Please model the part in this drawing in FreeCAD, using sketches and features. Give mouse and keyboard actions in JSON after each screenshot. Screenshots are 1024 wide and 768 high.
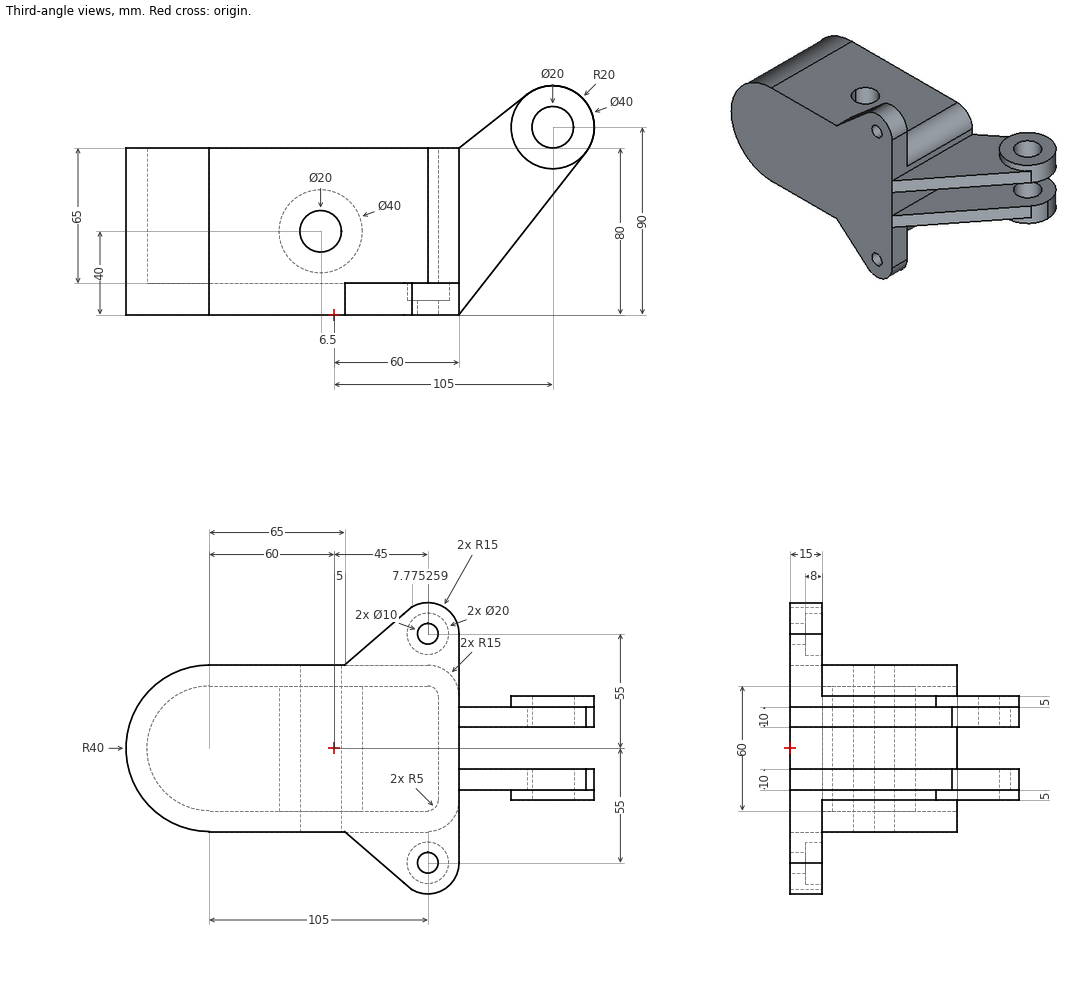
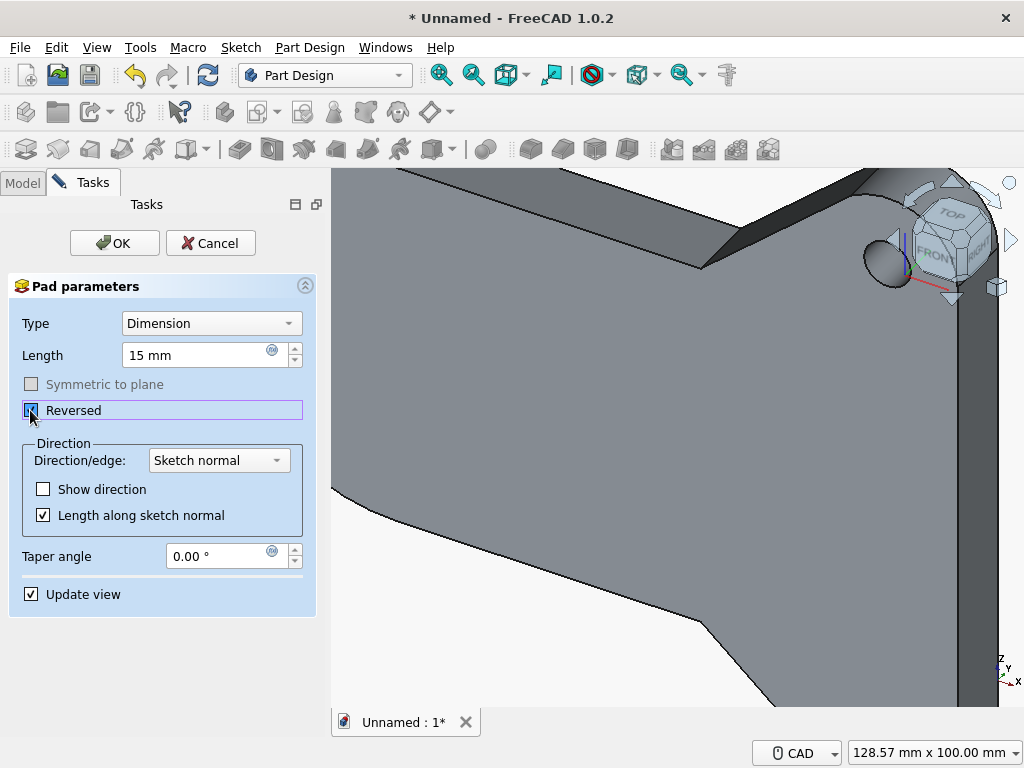
{"action": "left_click", "coordinate": [115, 243]}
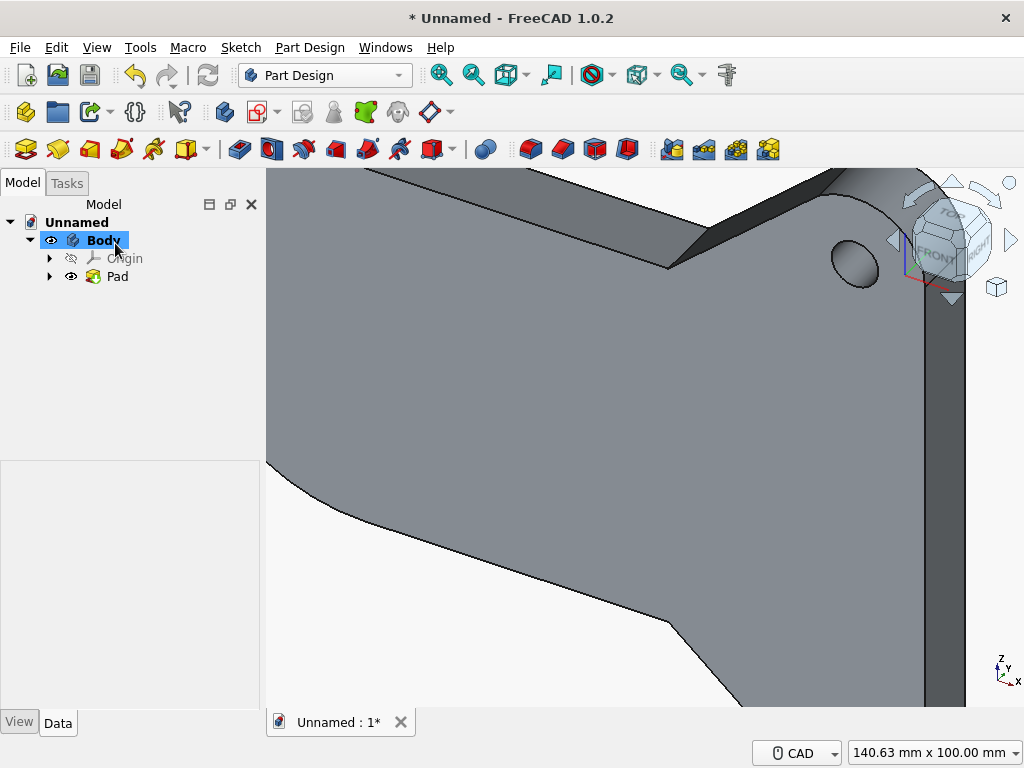
{"action": "left_click", "coordinate": [442, 76]}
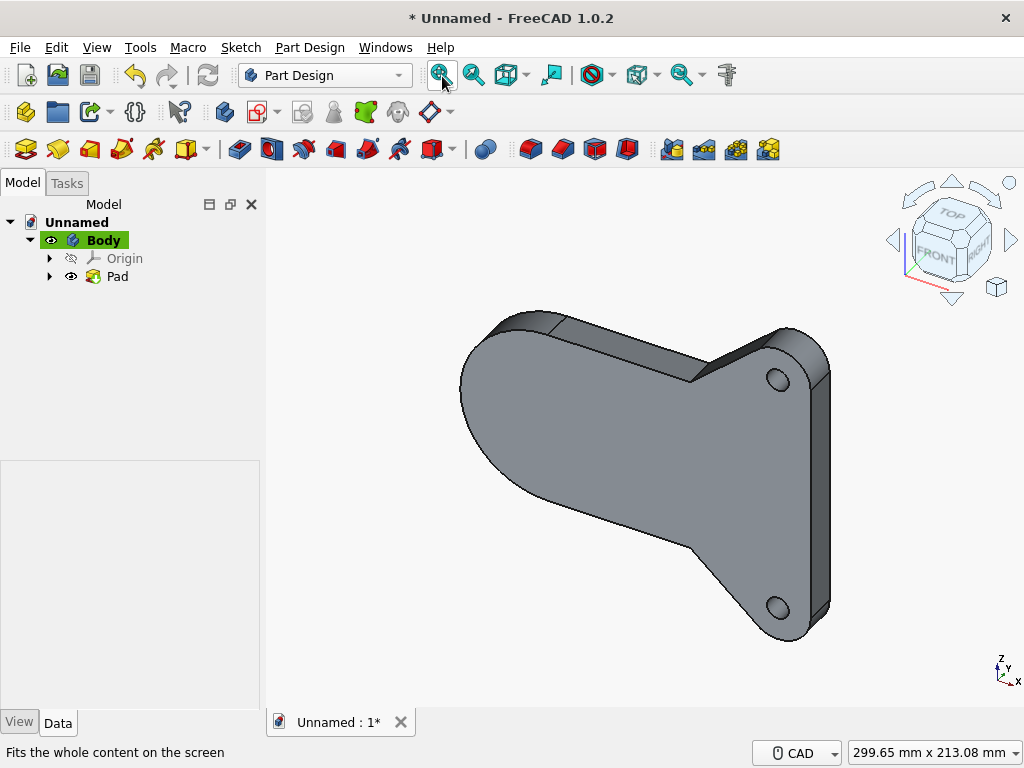
{"action": "key", "text": "4"}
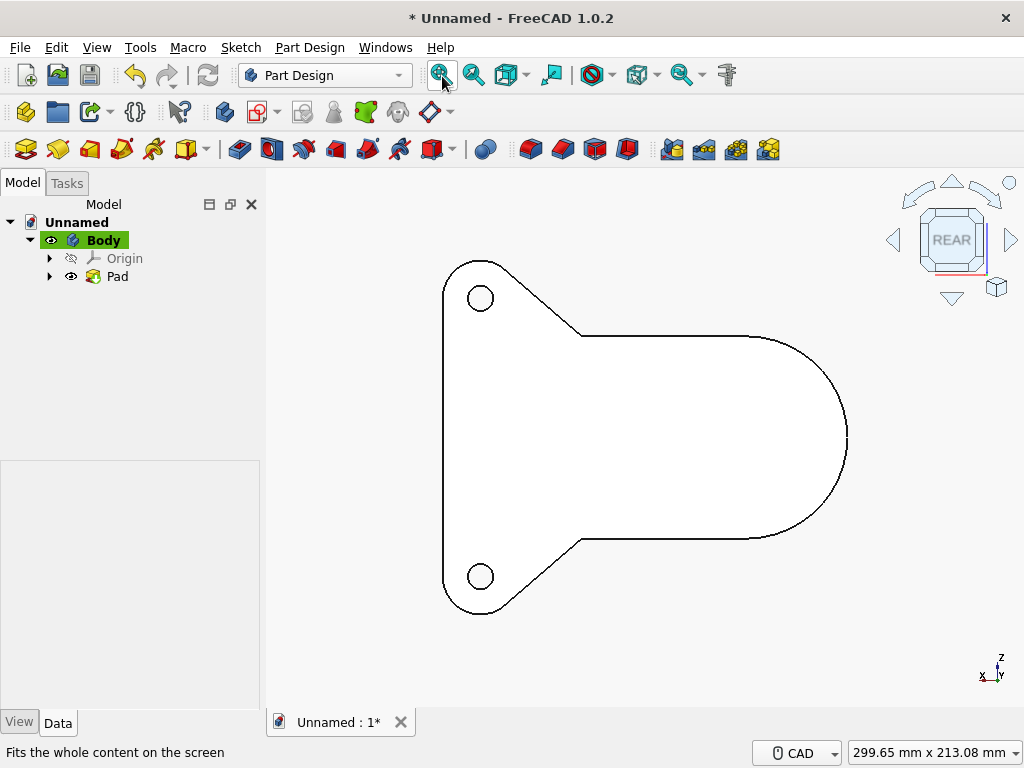
{"action": "left_click", "coordinate": [587, 436]}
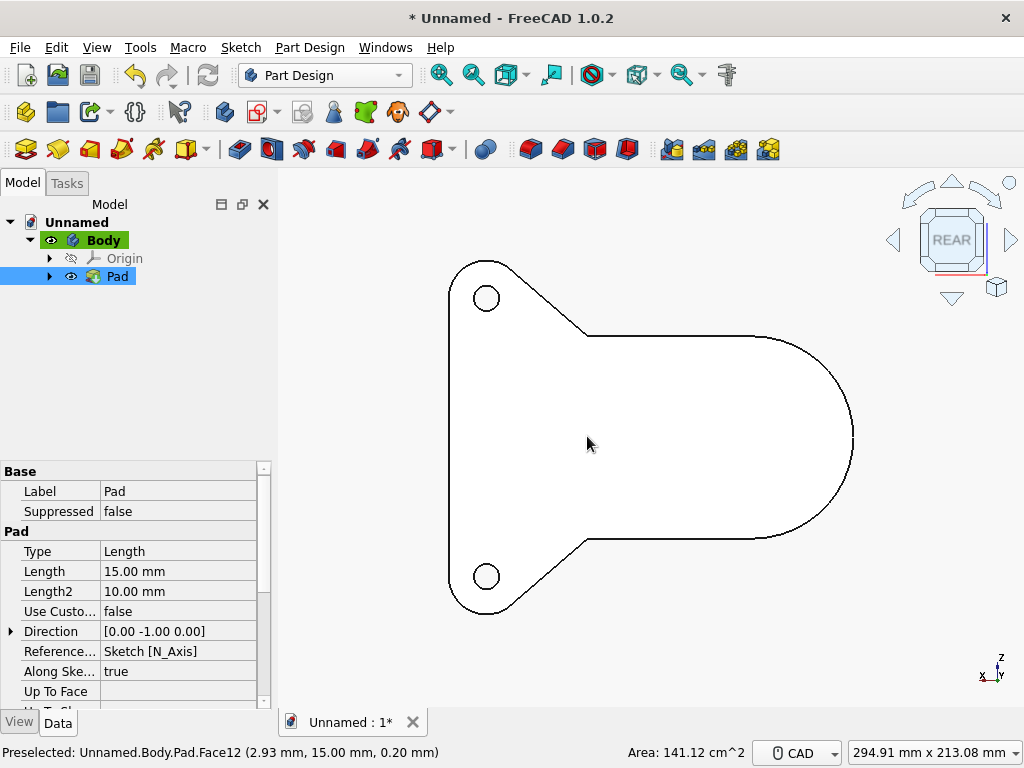
{"action": "left_click", "coordinate": [258, 112]}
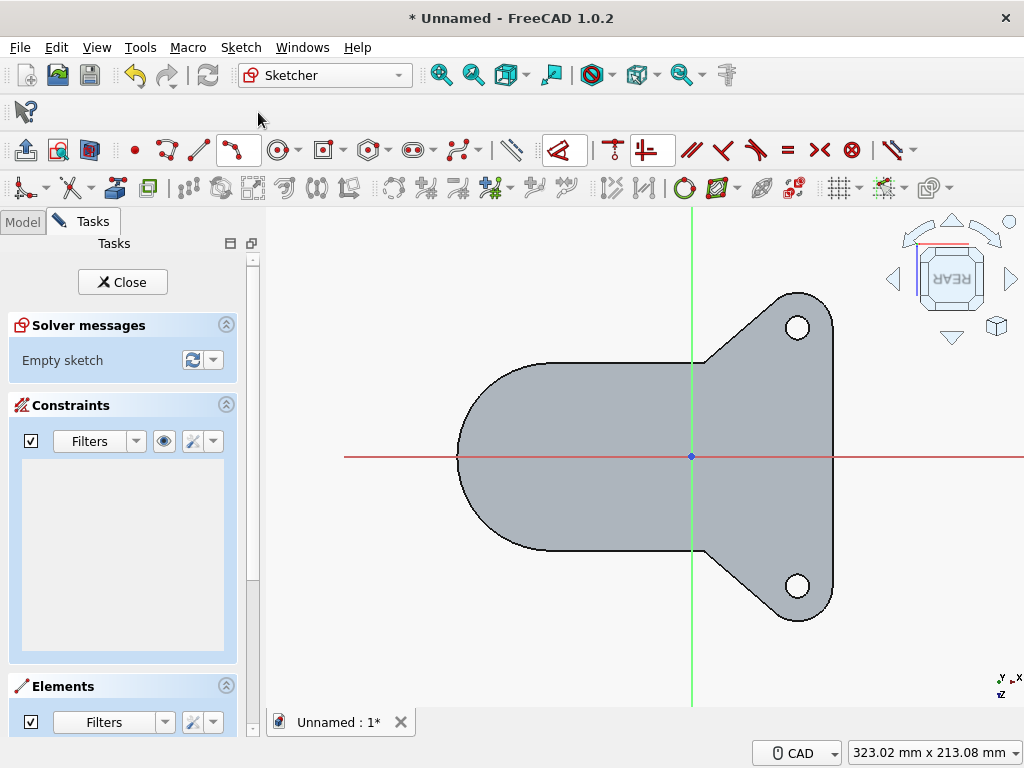
{"action": "left_click", "coordinate": [200, 150]}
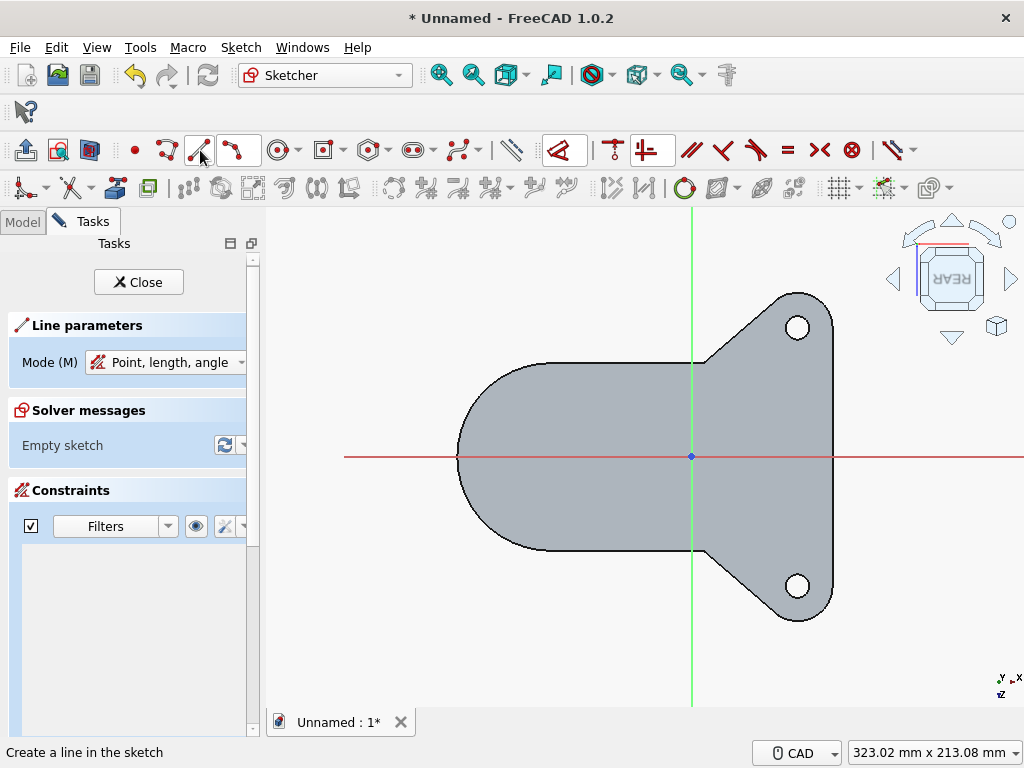
{"action": "left_click", "coordinate": [798, 363]}
{"action": "left_click", "coordinate": [551, 363]}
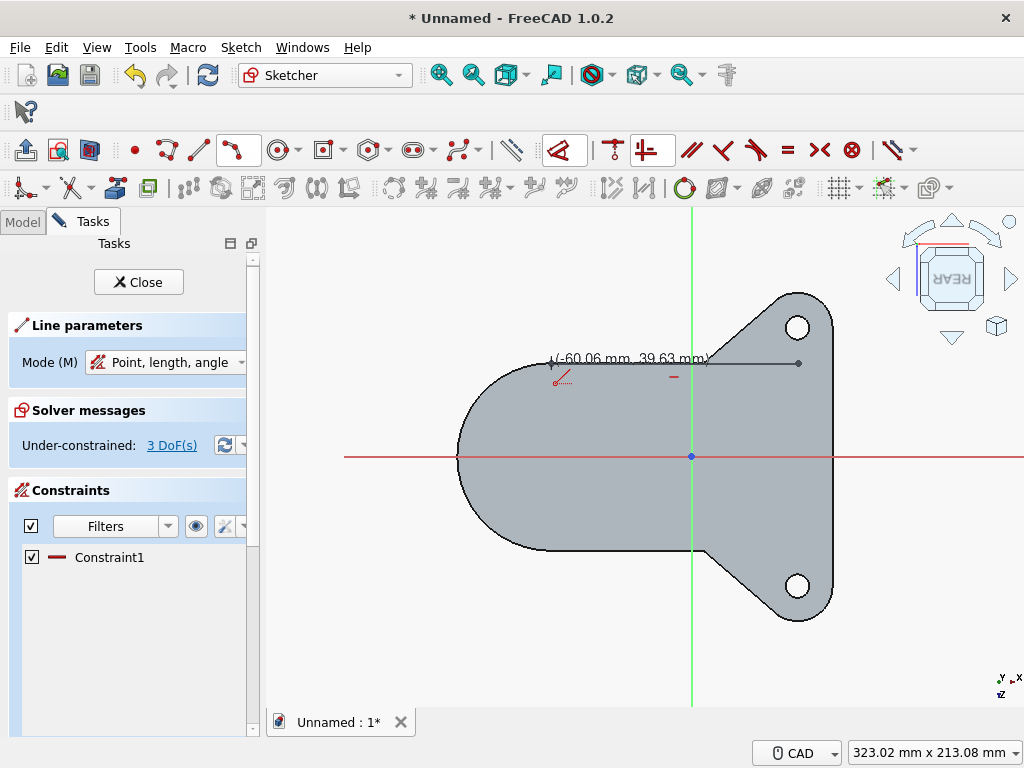
{"action": "left_click", "coordinate": [551, 551]}
{"action": "left_click", "coordinate": [798, 551]}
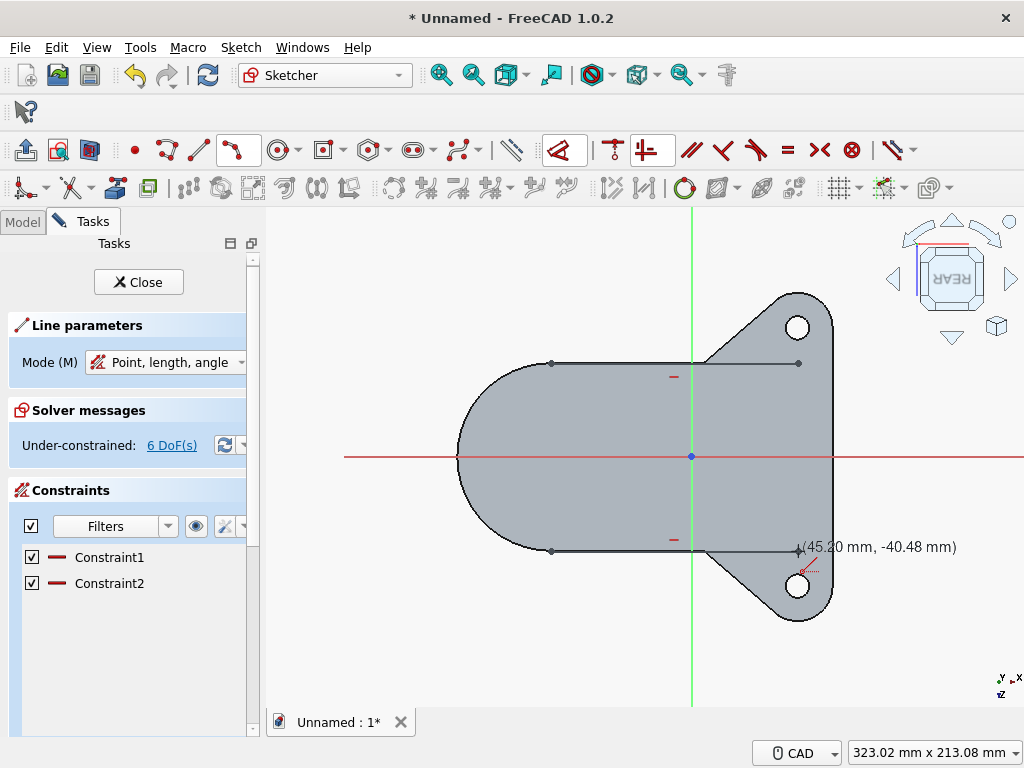
{"action": "left_click", "coordinate": [833, 516]}
{"action": "left_click", "coordinate": [833, 398]}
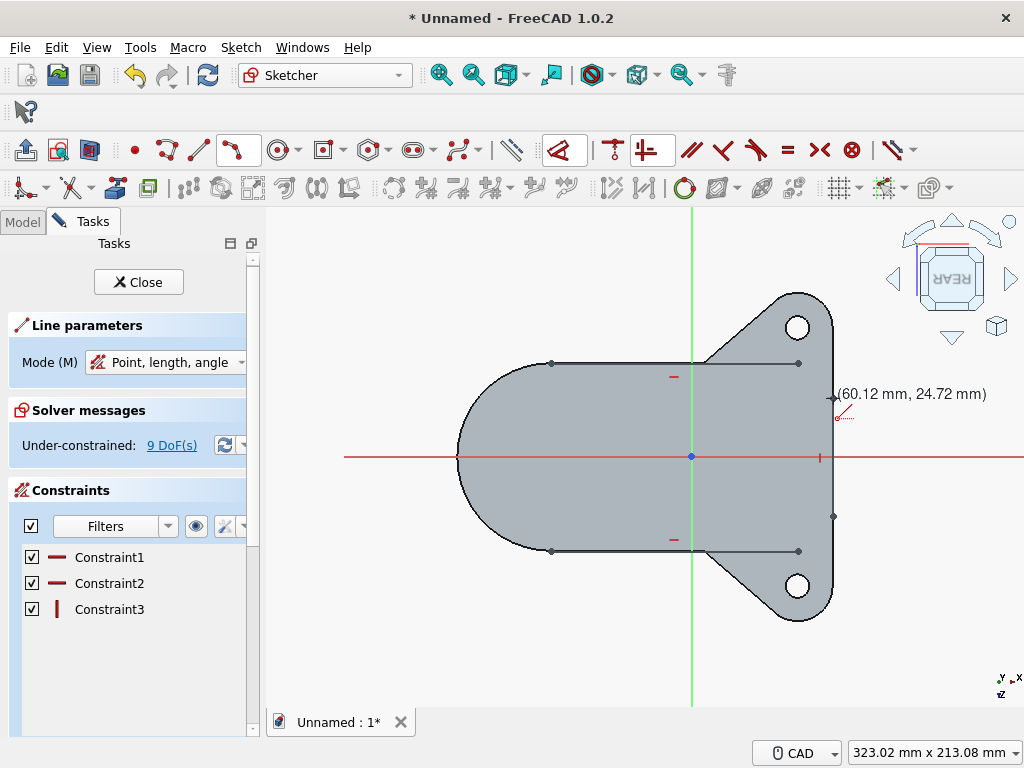
{"action": "left_click", "coordinate": [232, 150]}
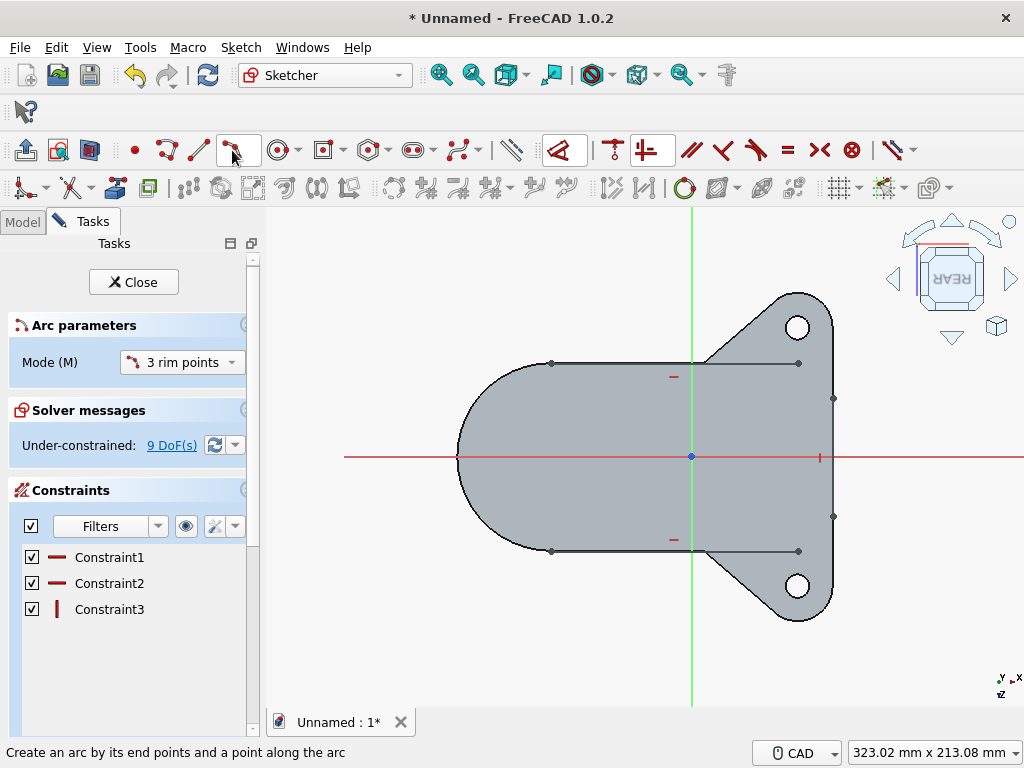
{"action": "left_click", "coordinate": [551, 364]}
{"action": "left_click", "coordinate": [551, 552]}
{"action": "left_click", "coordinate": [462, 428]}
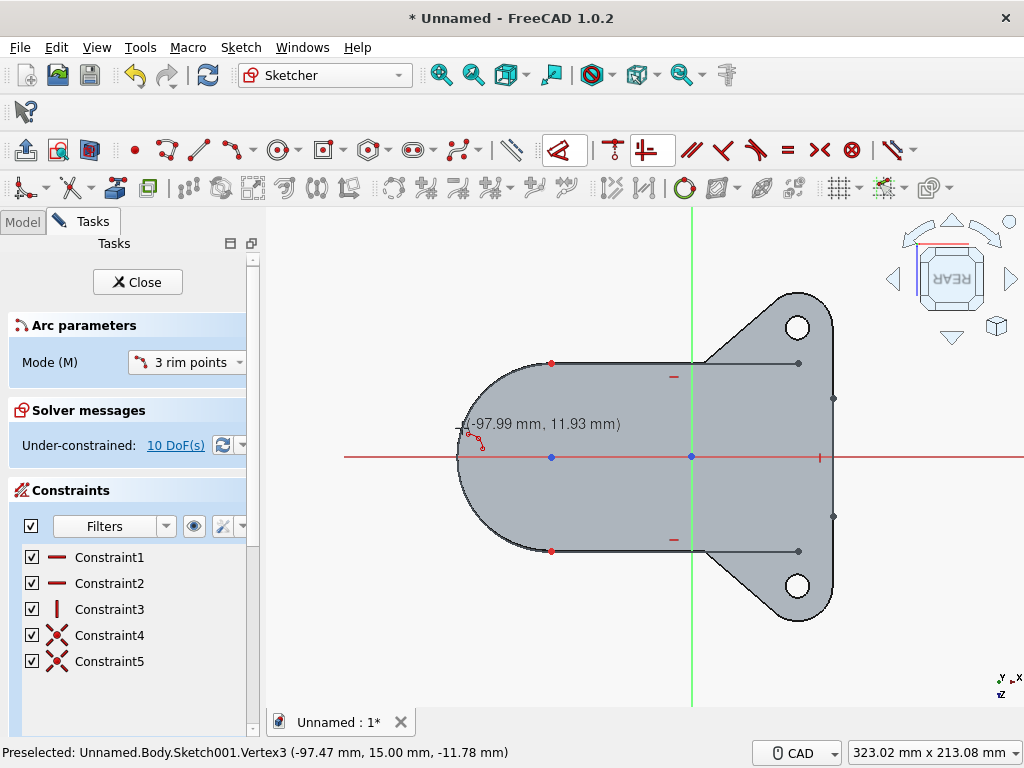
{"action": "left_click", "coordinate": [798, 552]}
{"action": "left_click", "coordinate": [833, 517]}